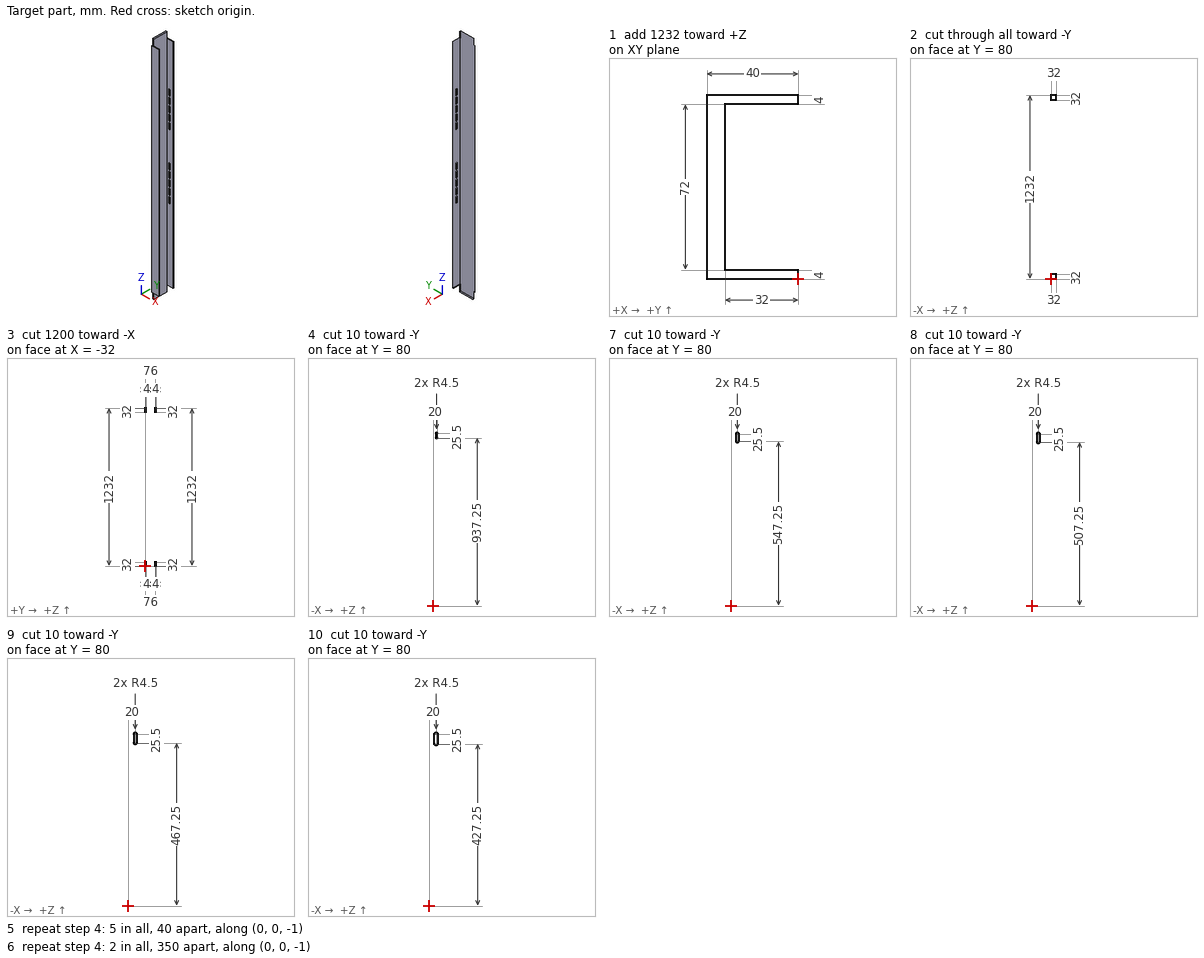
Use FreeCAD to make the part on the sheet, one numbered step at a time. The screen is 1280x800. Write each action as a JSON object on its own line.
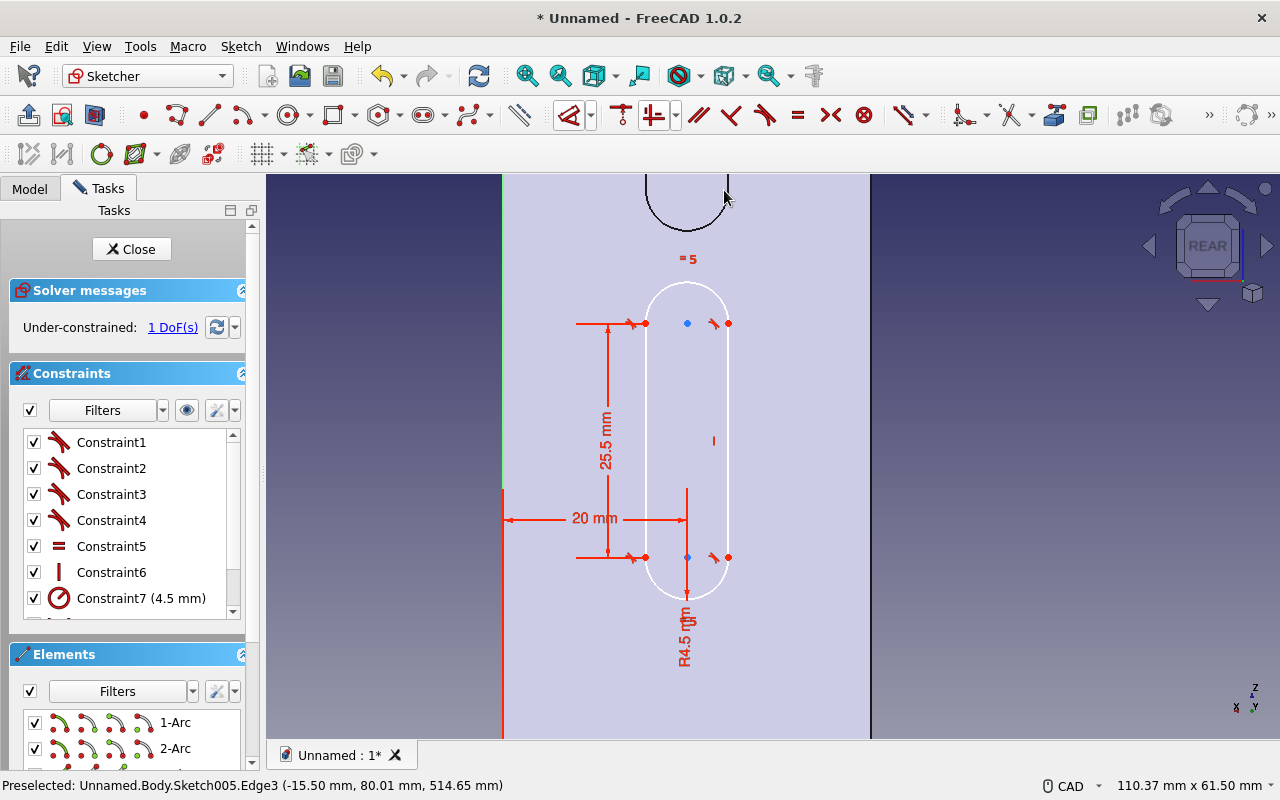
{"action": "left_click", "coordinate": [646, 558]}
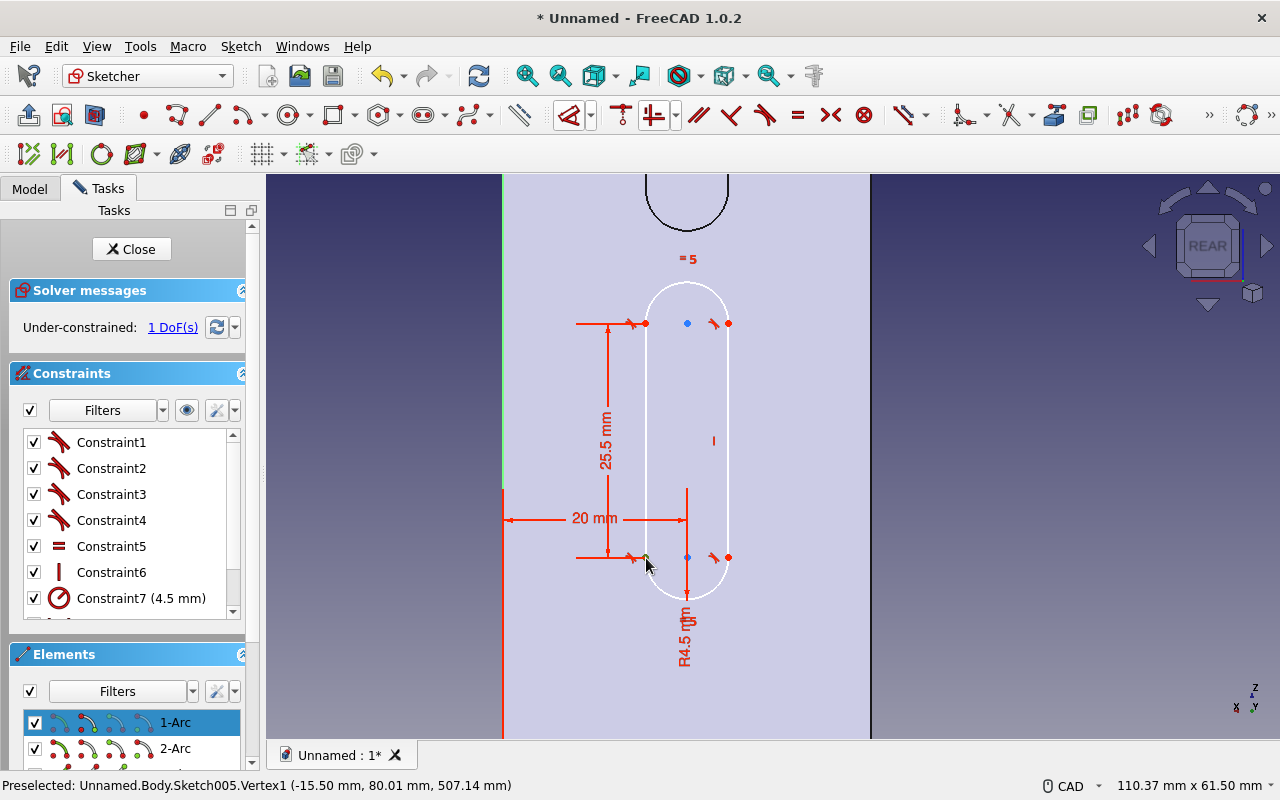
{"action": "key", "text": "i"}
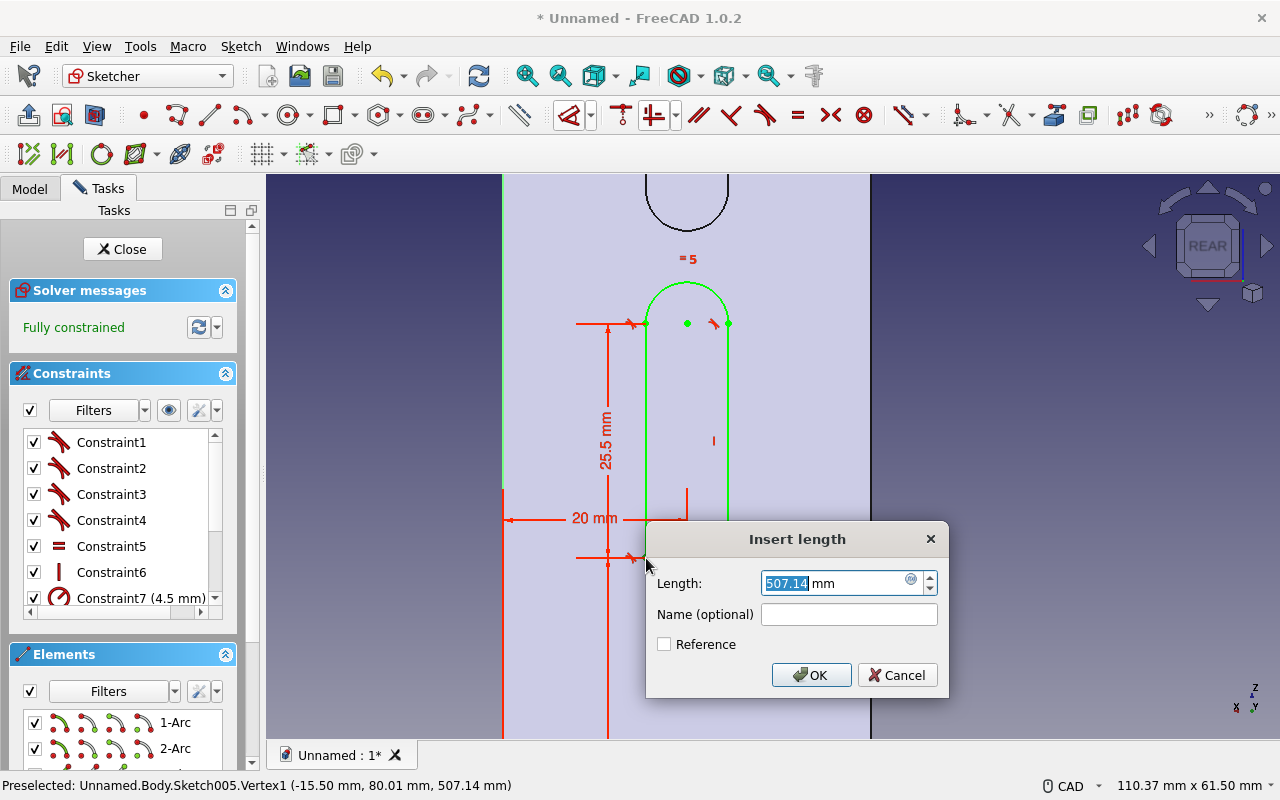
{"action": "type", "text": "507.25"}
{"action": "key", "text": "Return"}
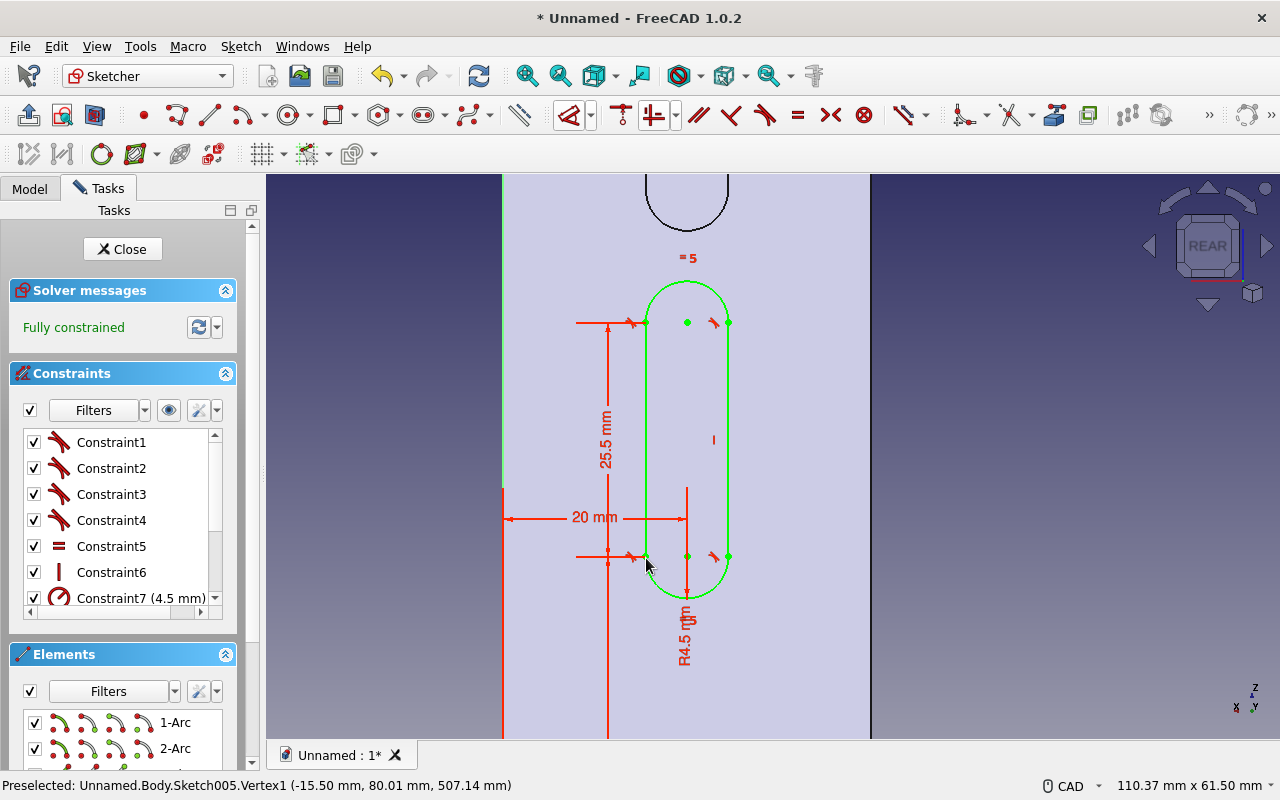
{"action": "left_click", "coordinate": [123, 249]}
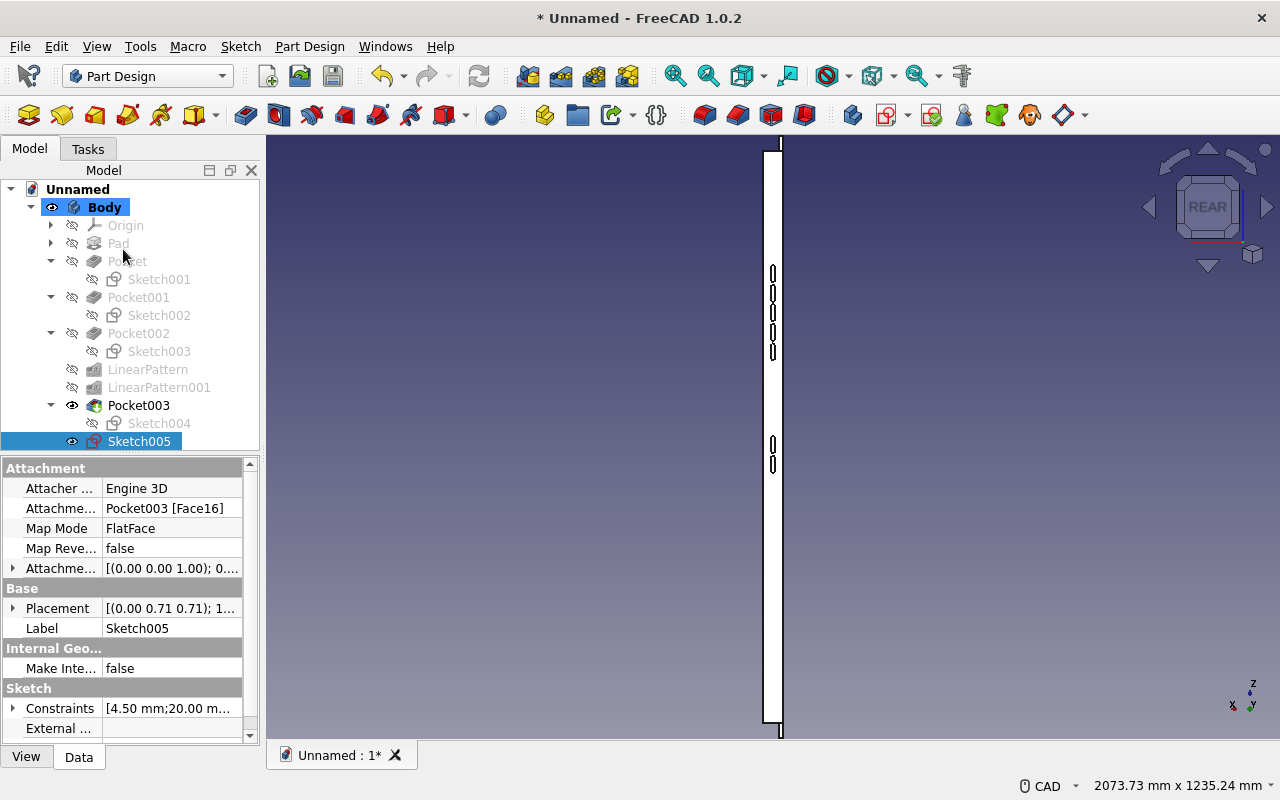
{"action": "left_click", "coordinate": [246, 116]}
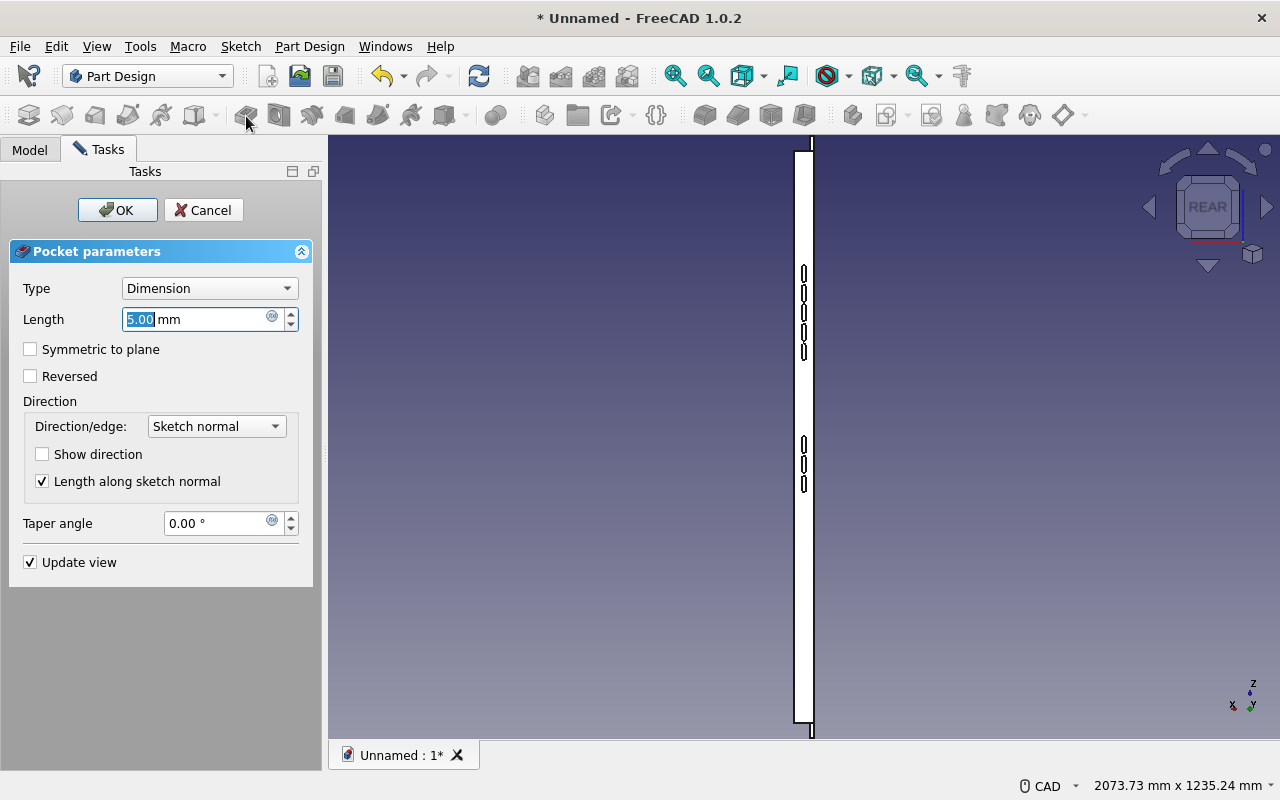
{"action": "type", "text": "10"}
{"action": "key", "text": "Tab"}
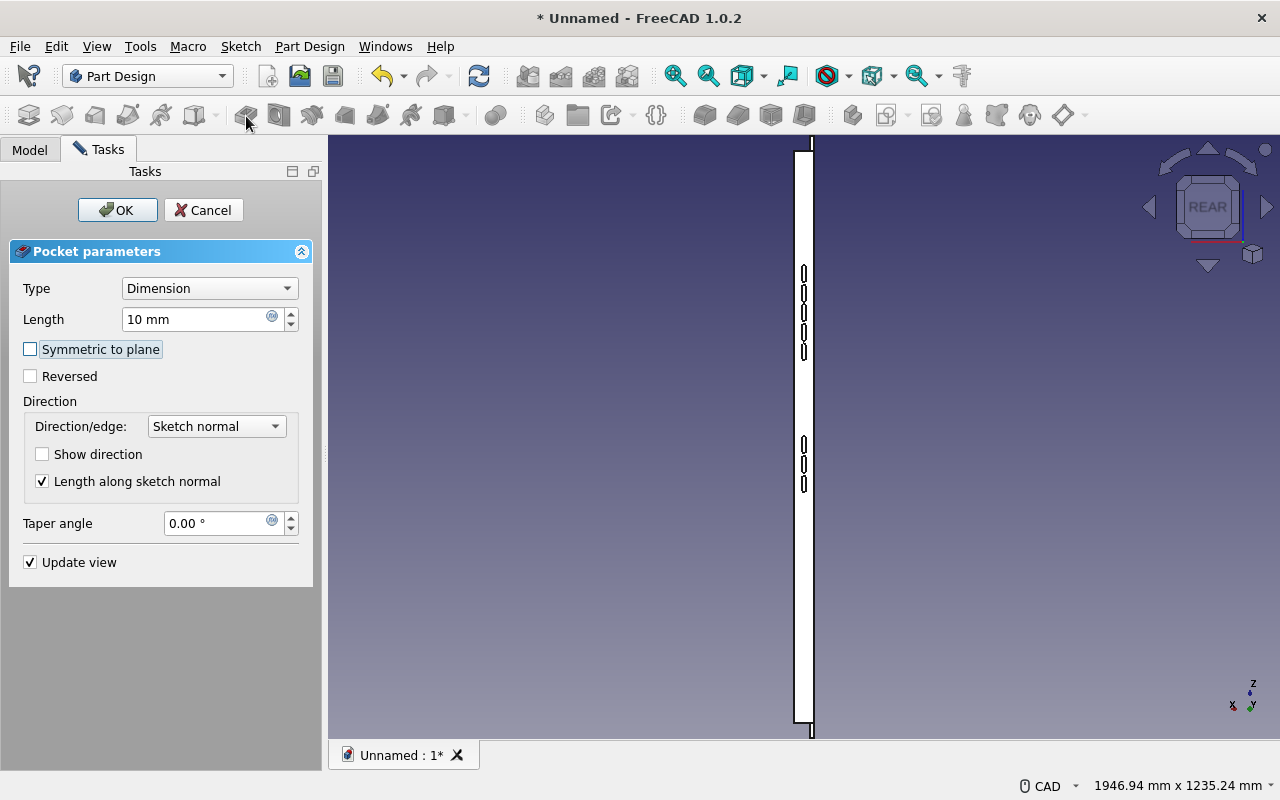
{"action": "left_click", "coordinate": [118, 210]}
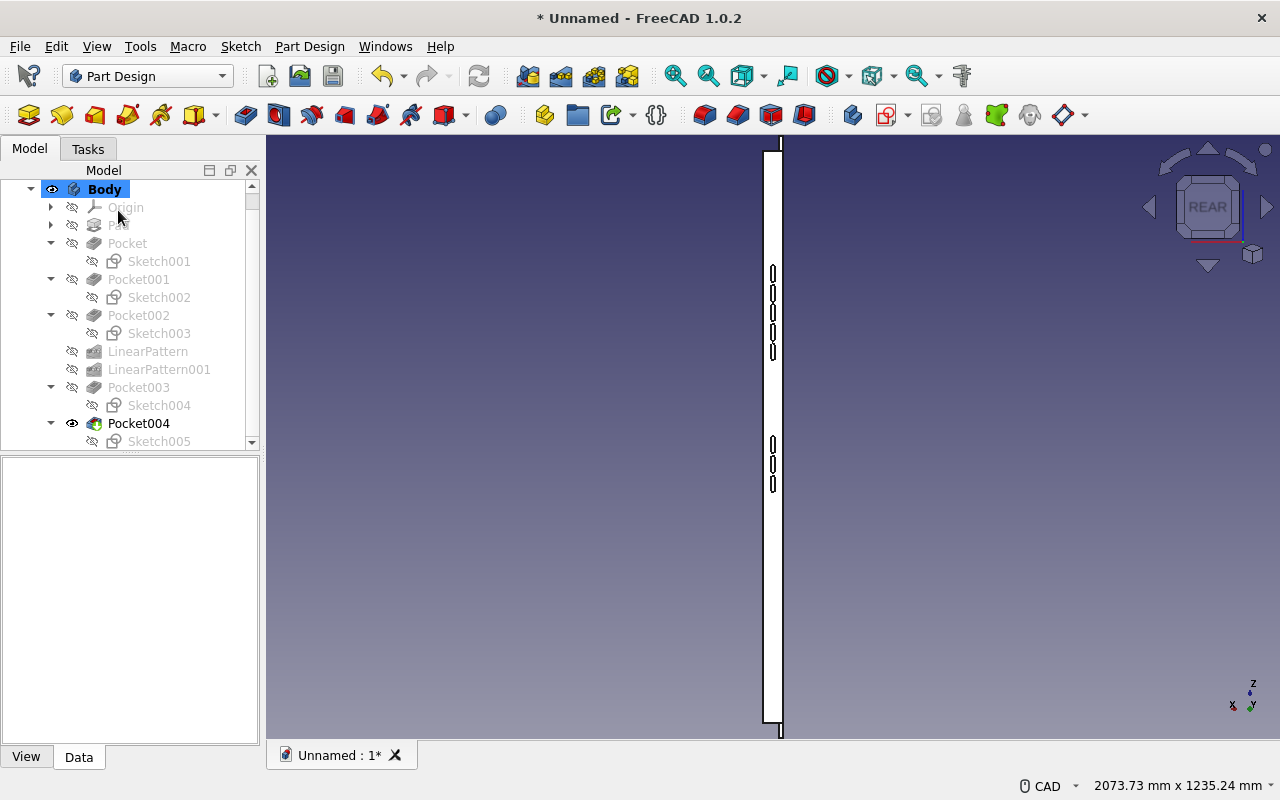
{"action": "left_click", "coordinate": [773, 191]}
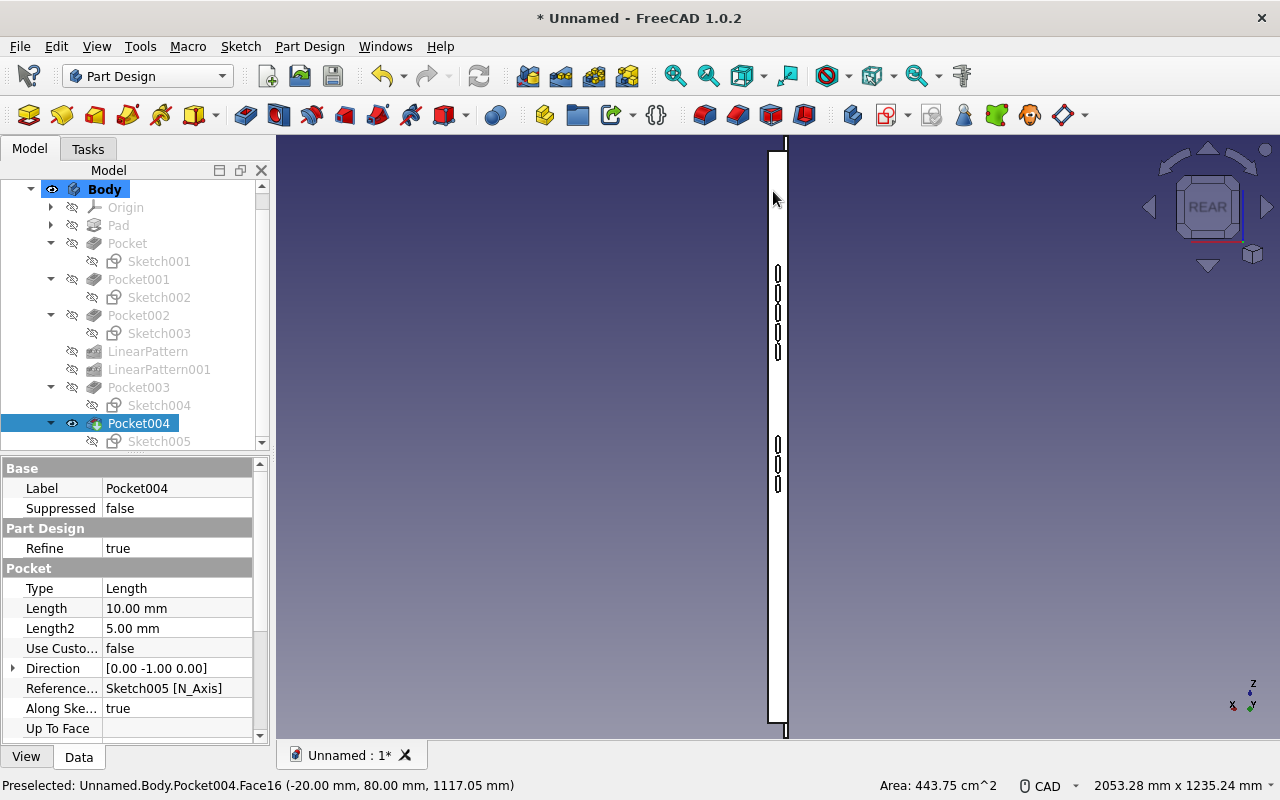
{"action": "left_click", "coordinate": [886, 116]}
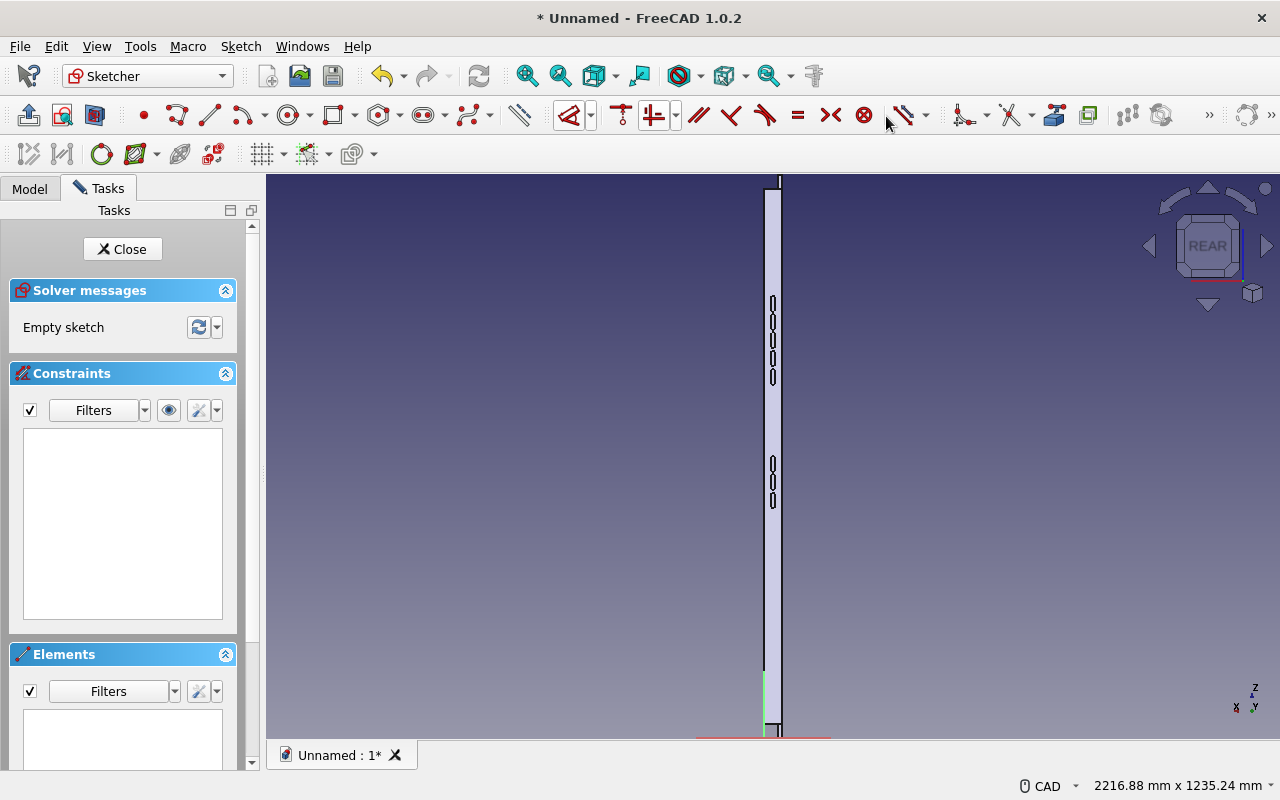
{"action": "scroll", "coordinate": [777, 522], "scroll_direction": "up", "scroll_amount": 15}